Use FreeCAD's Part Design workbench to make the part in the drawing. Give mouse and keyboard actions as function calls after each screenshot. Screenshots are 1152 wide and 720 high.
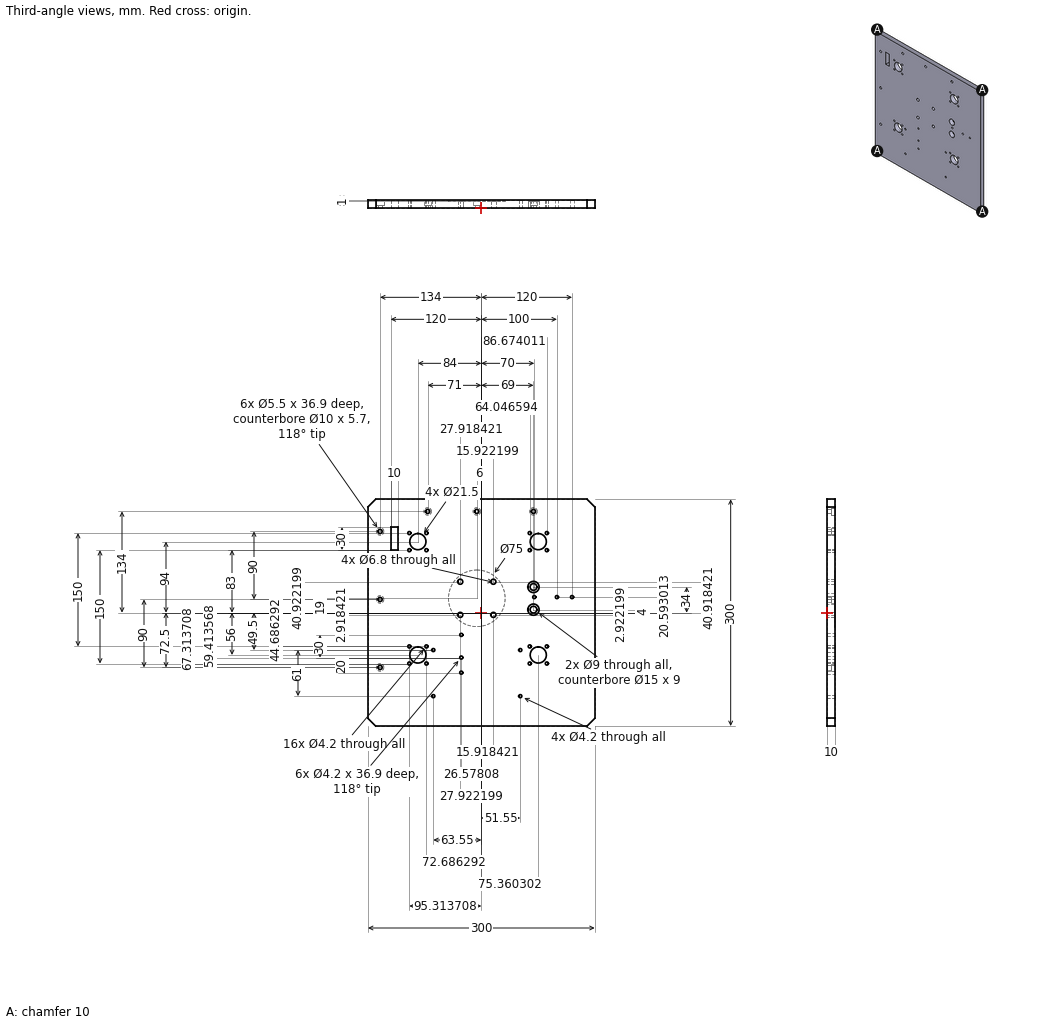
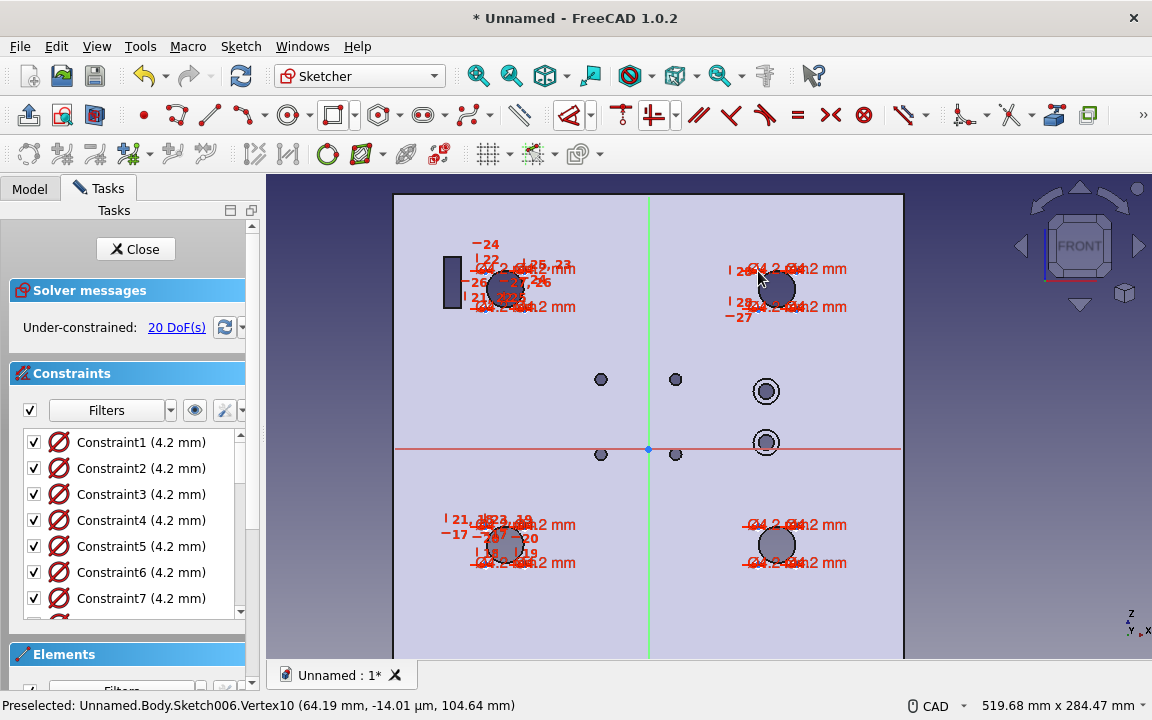
click(525, 271)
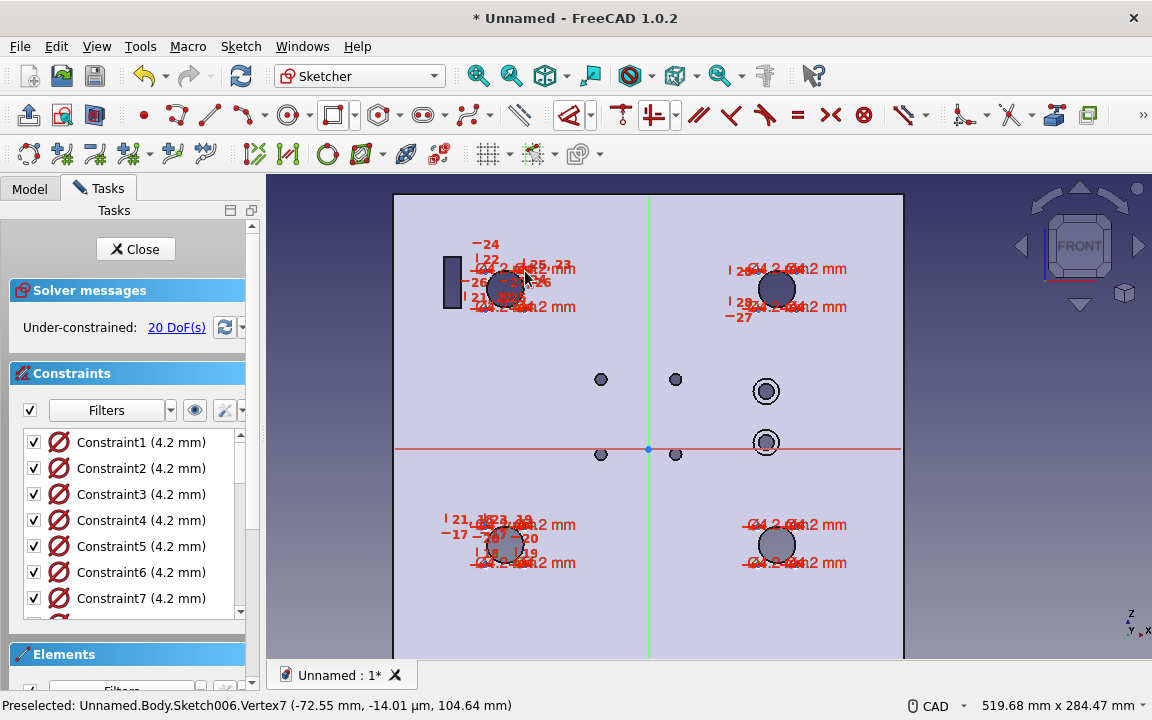
click(758, 271)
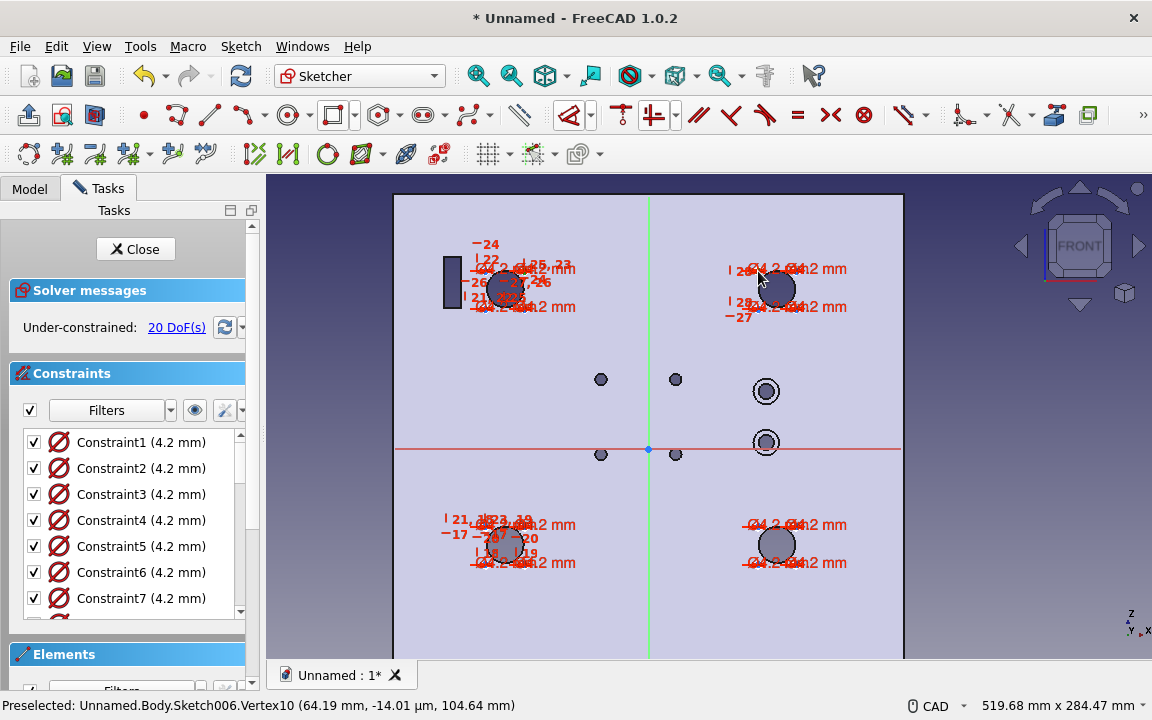
key(h)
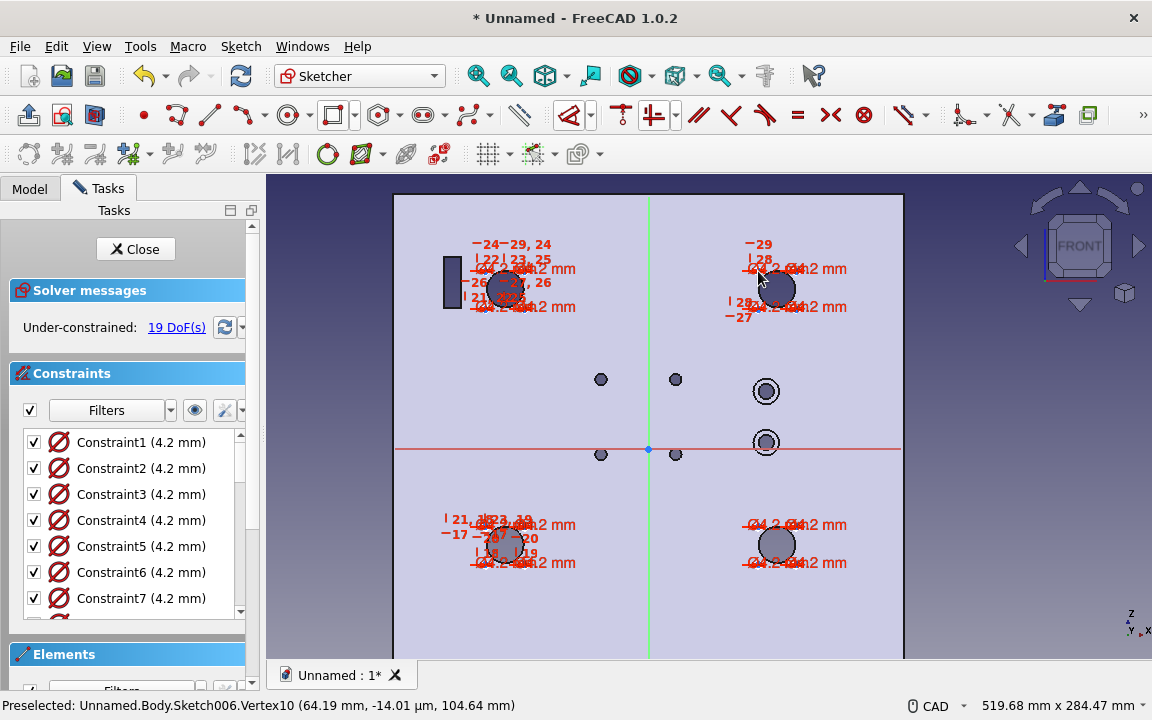
click(758, 271)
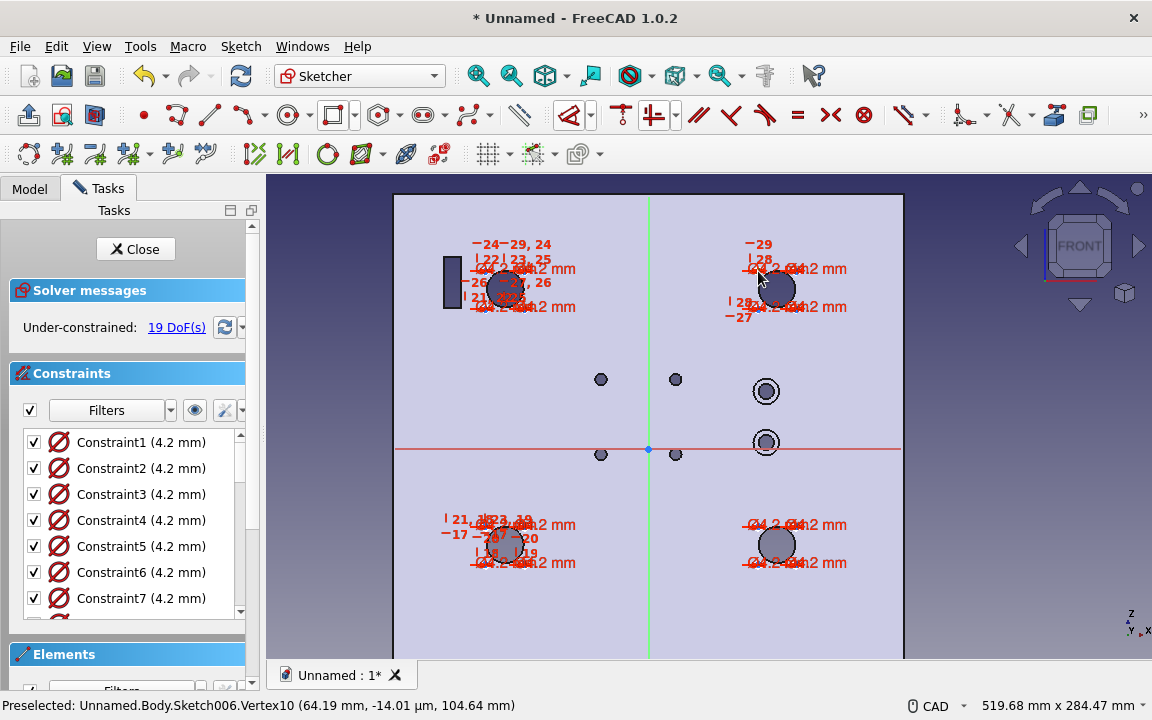
click(796, 271)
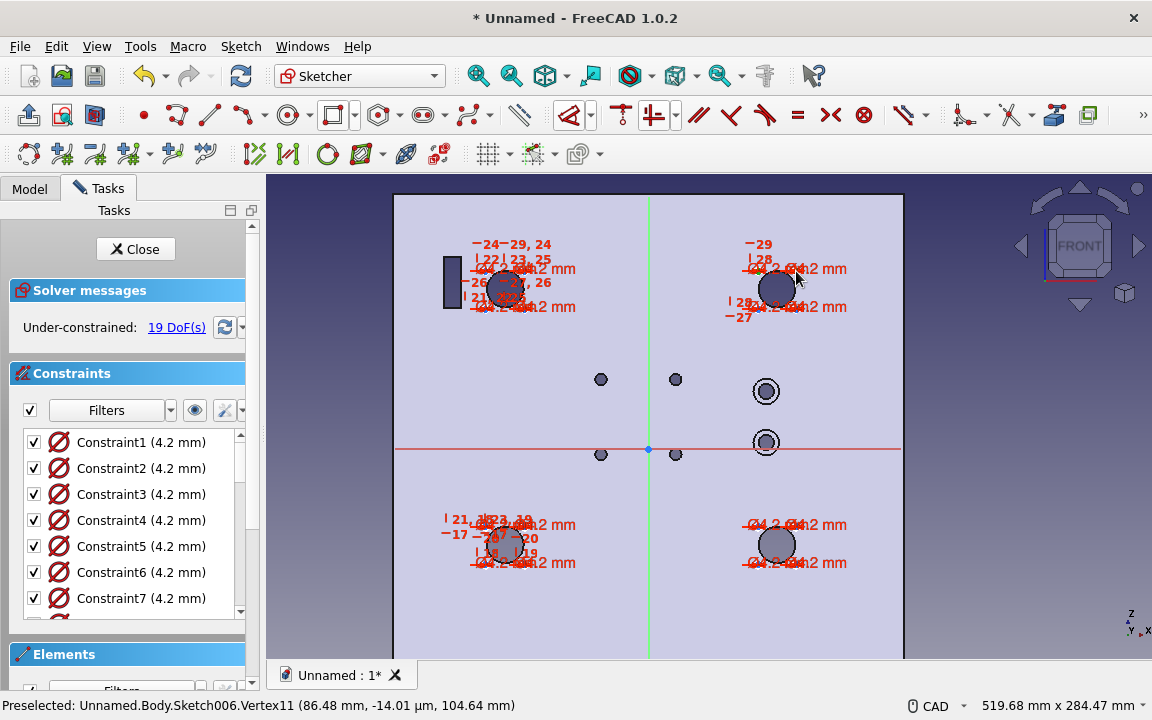
key(h)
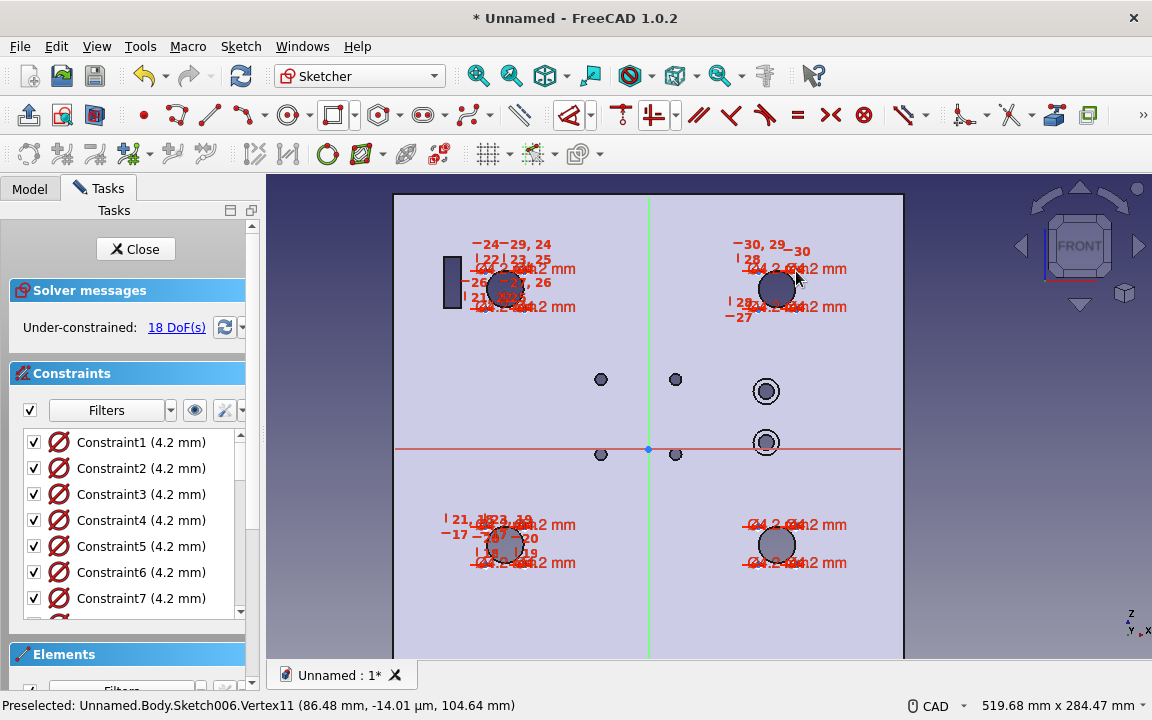
click(796, 271)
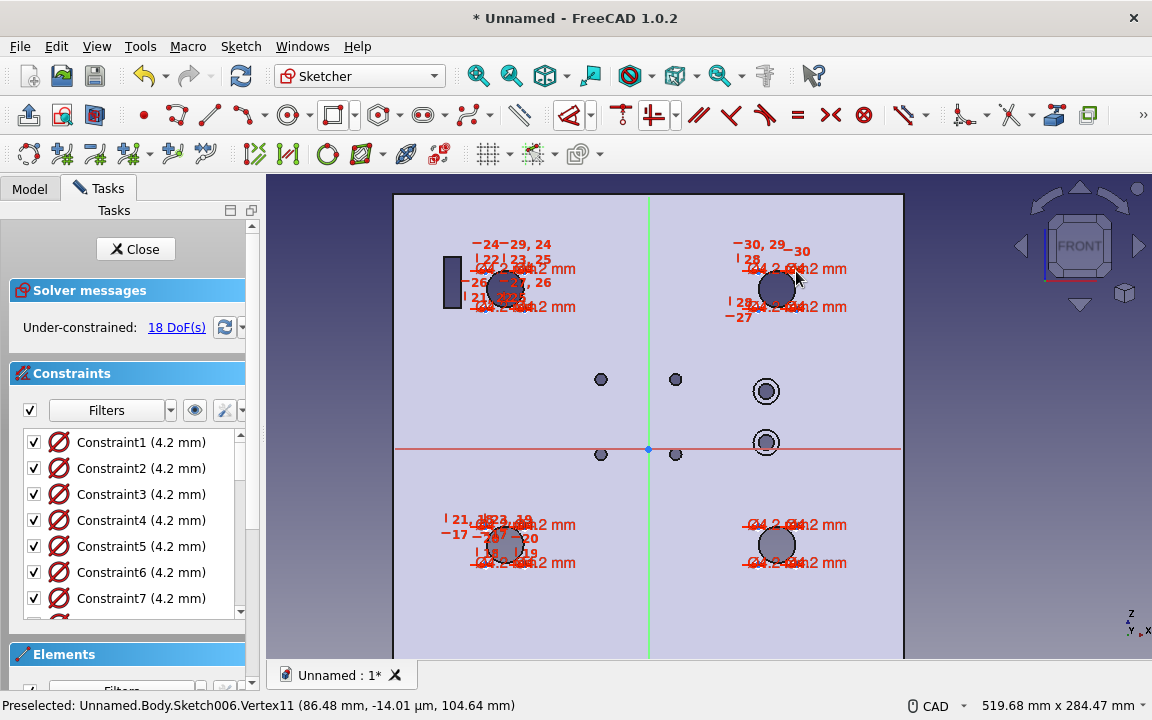
click(796, 309)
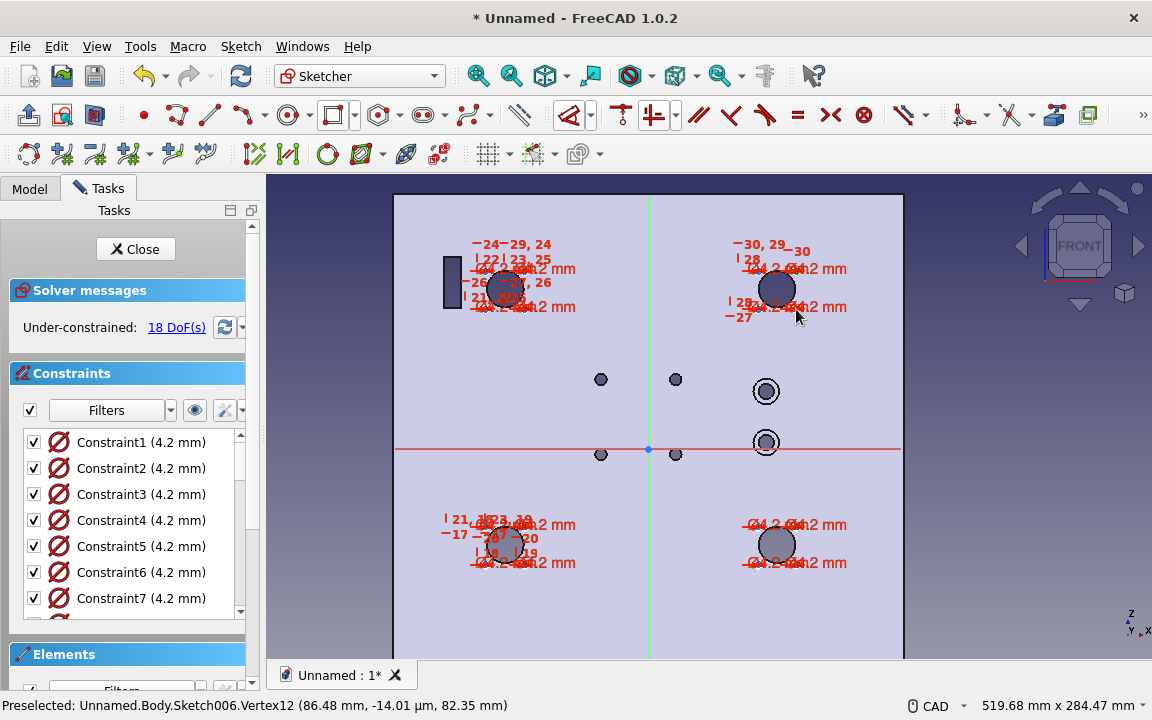
click(676, 116)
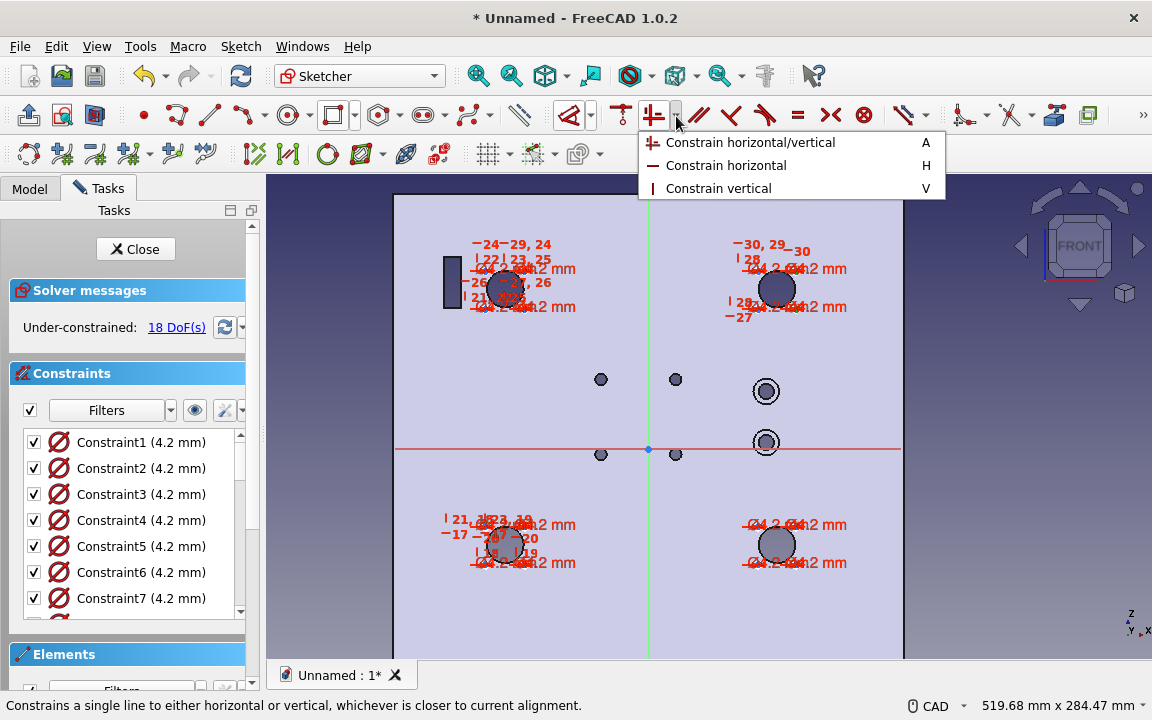
click(792, 188)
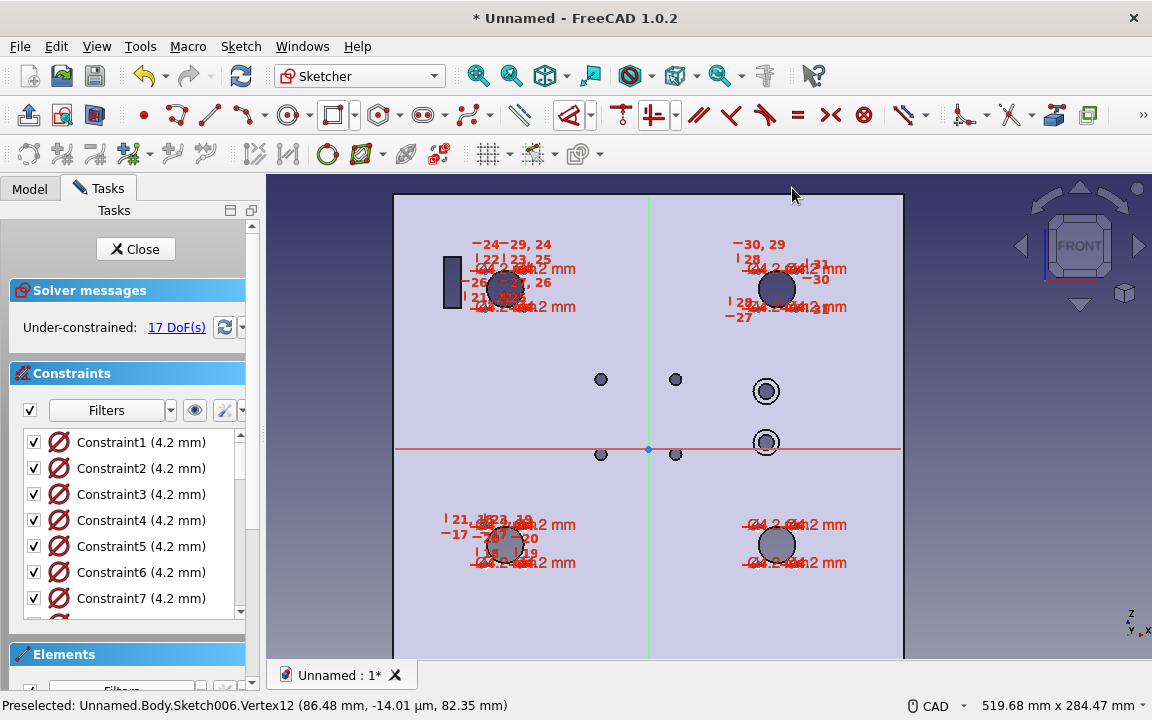
click(758, 309)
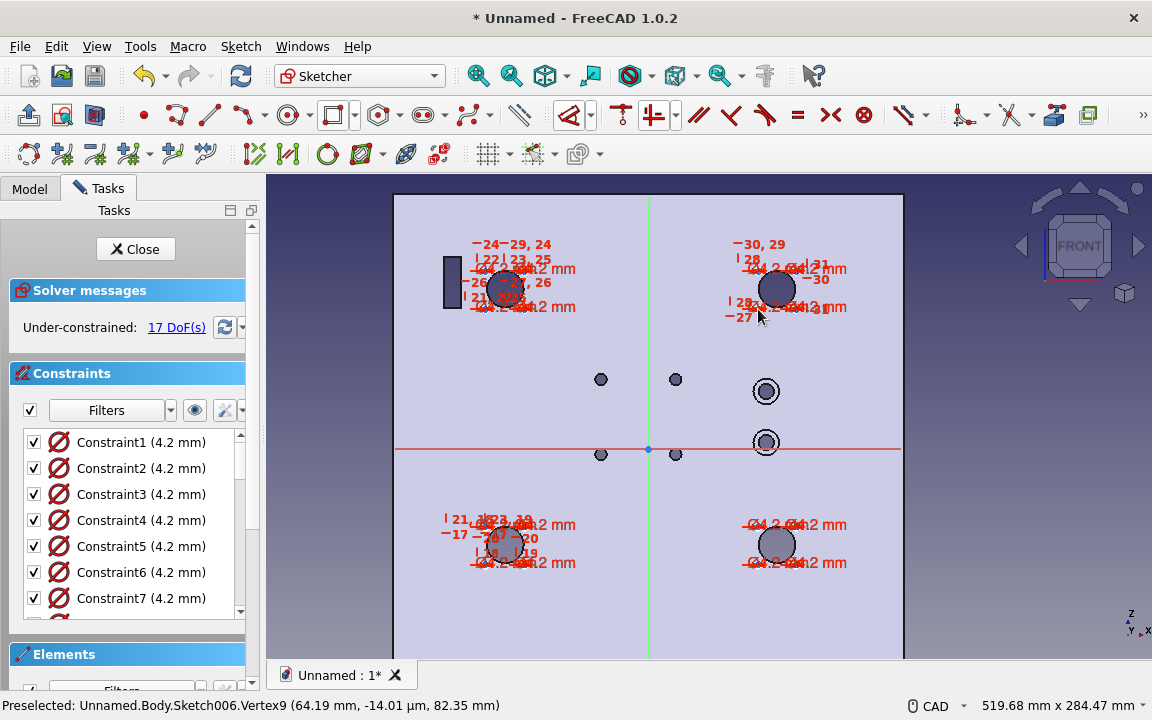
click(796, 309)